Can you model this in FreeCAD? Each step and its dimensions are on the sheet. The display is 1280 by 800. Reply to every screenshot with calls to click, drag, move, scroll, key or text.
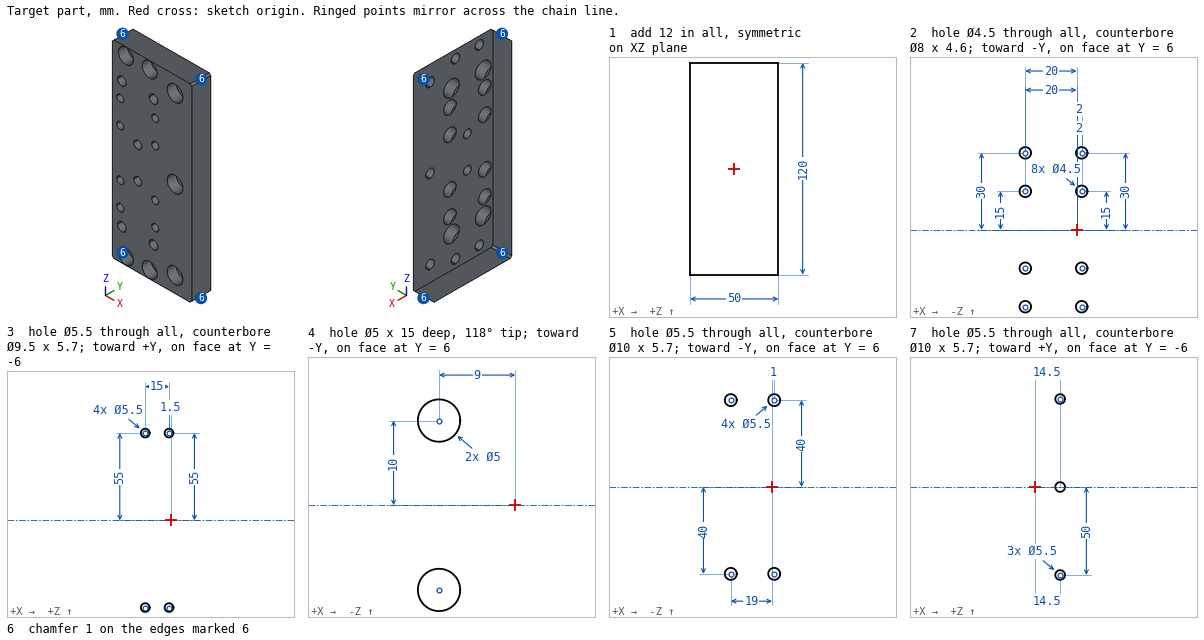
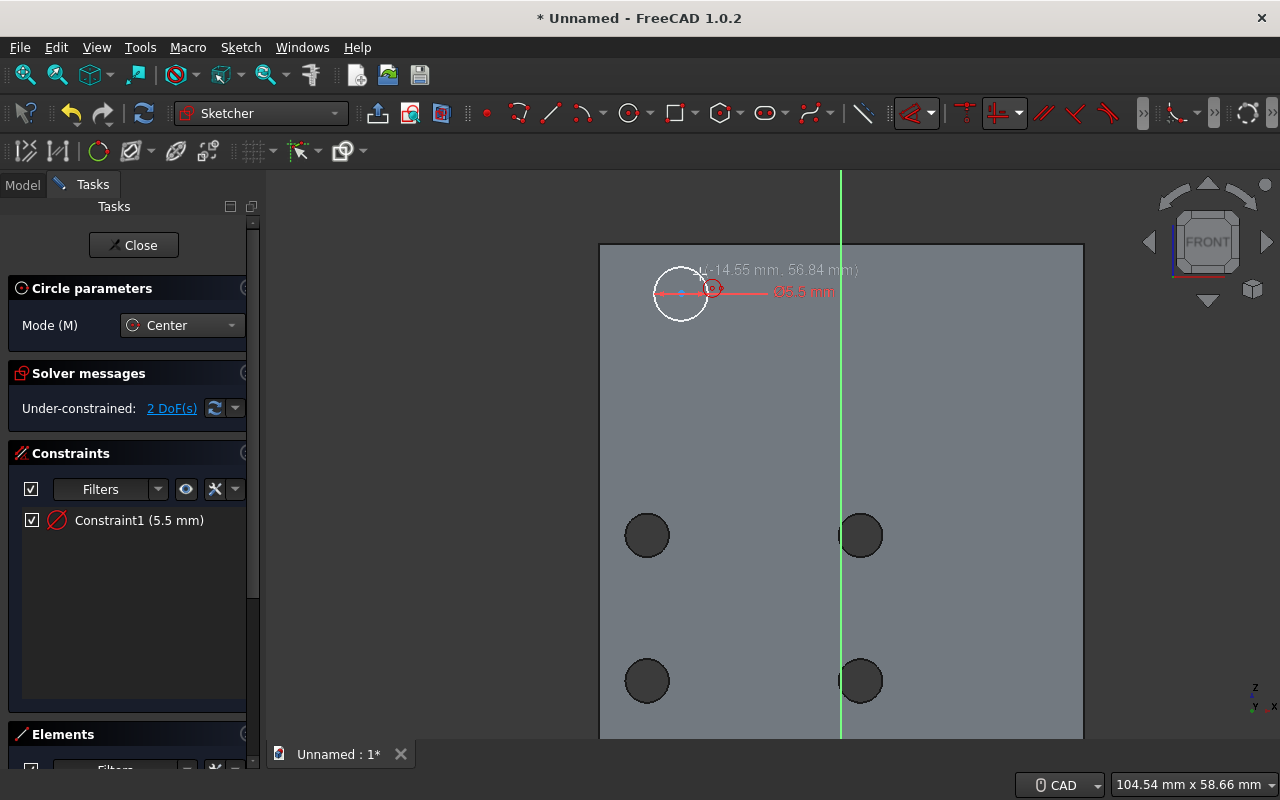
click(827, 293)
move(808, 274)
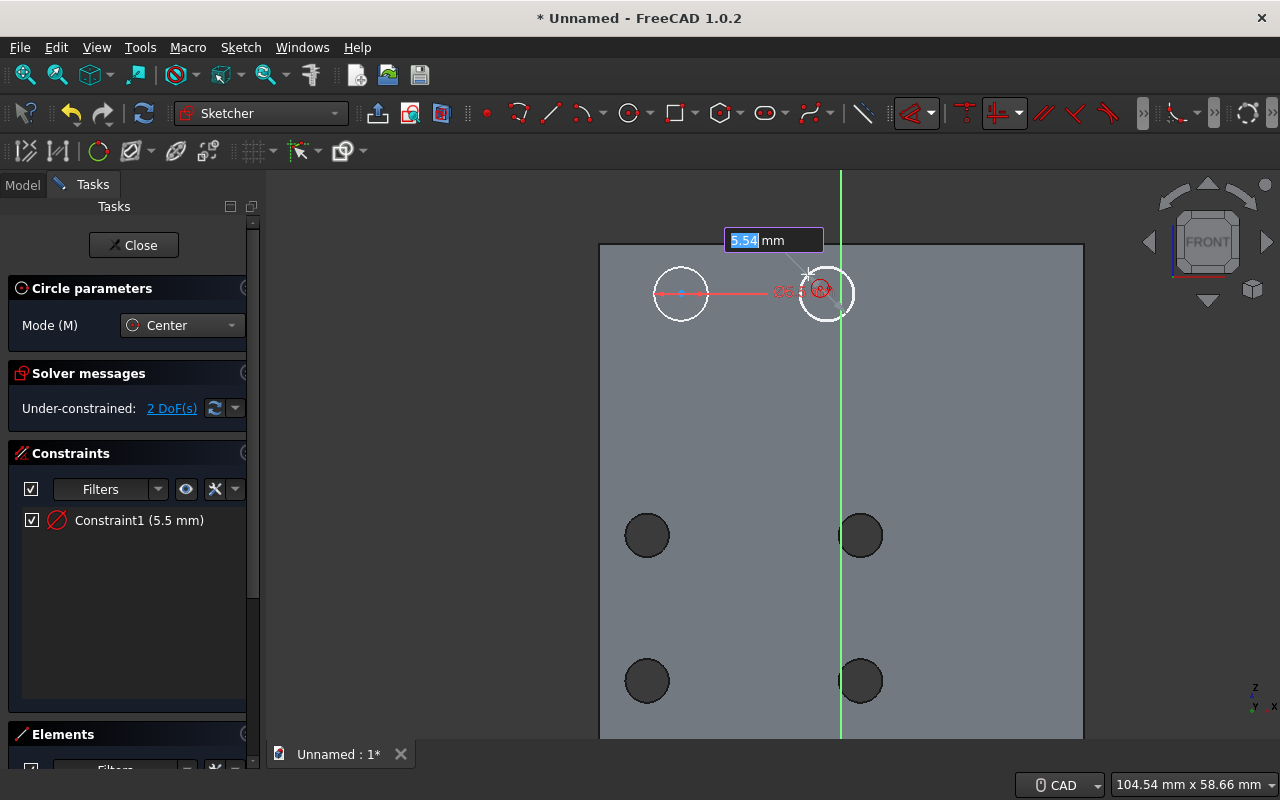
text(5.5)
key(Return)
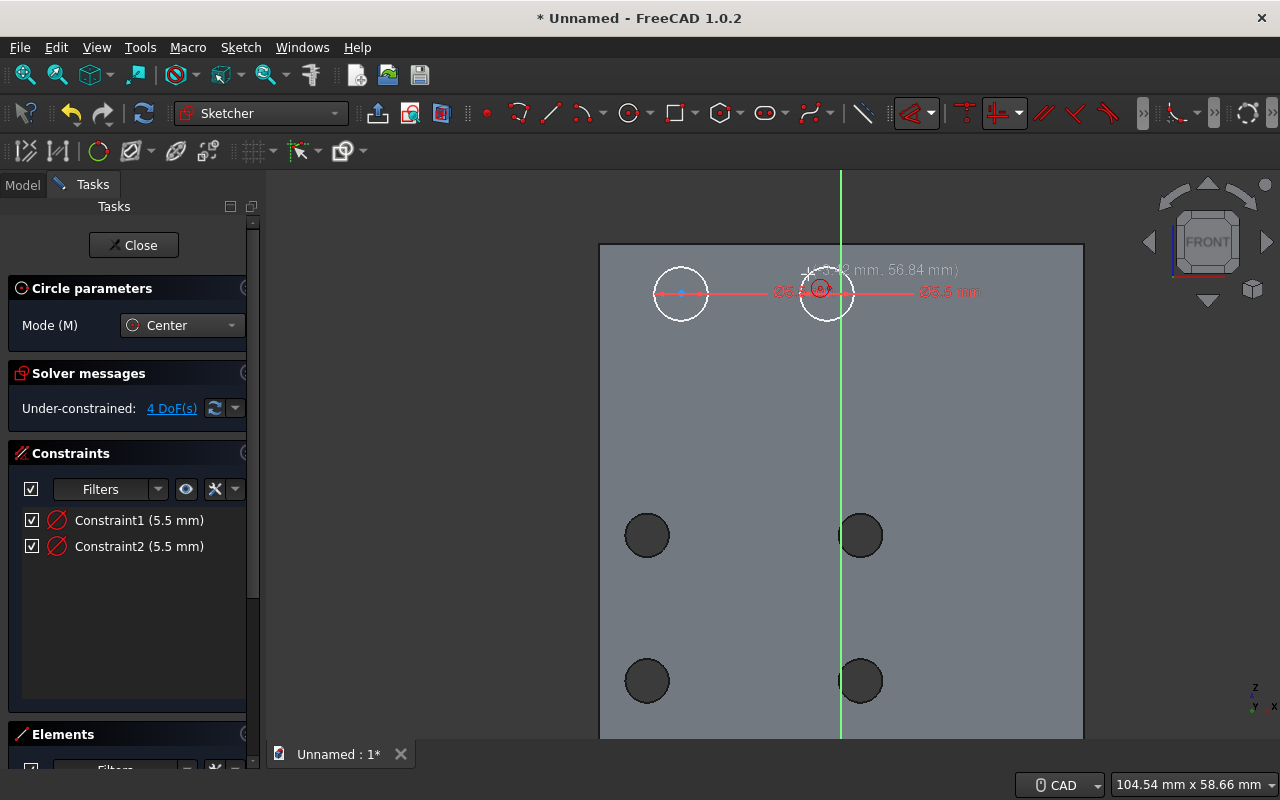
scroll(683, 294, down, 6)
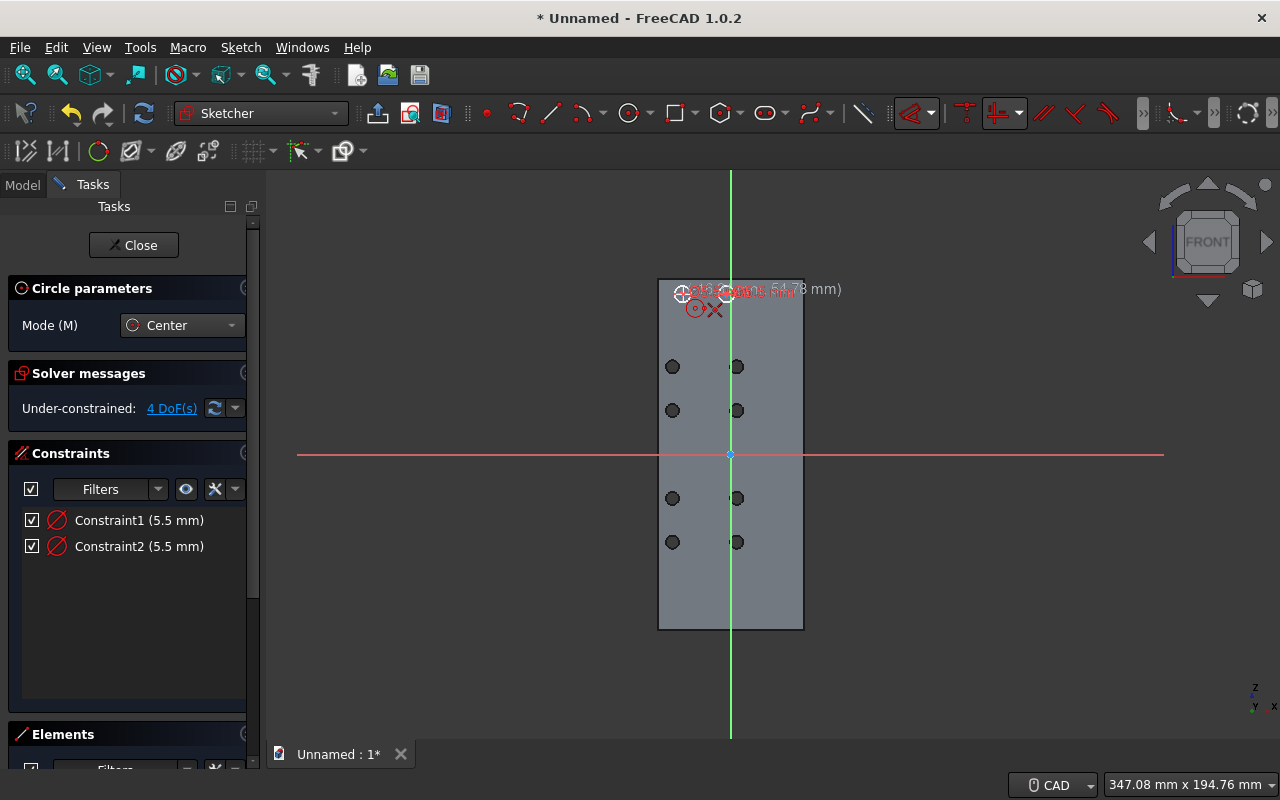
scroll(727, 615, up, 7)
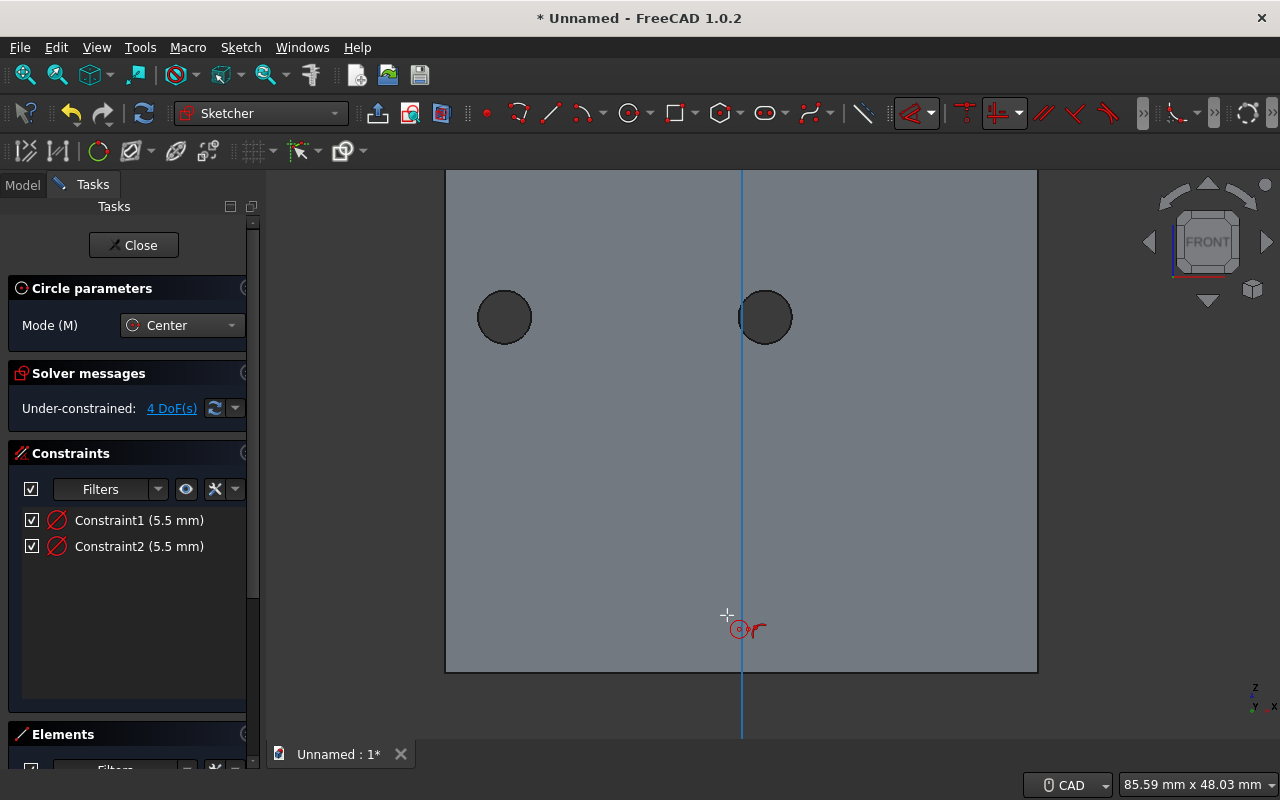
click(724, 613)
move(701, 590)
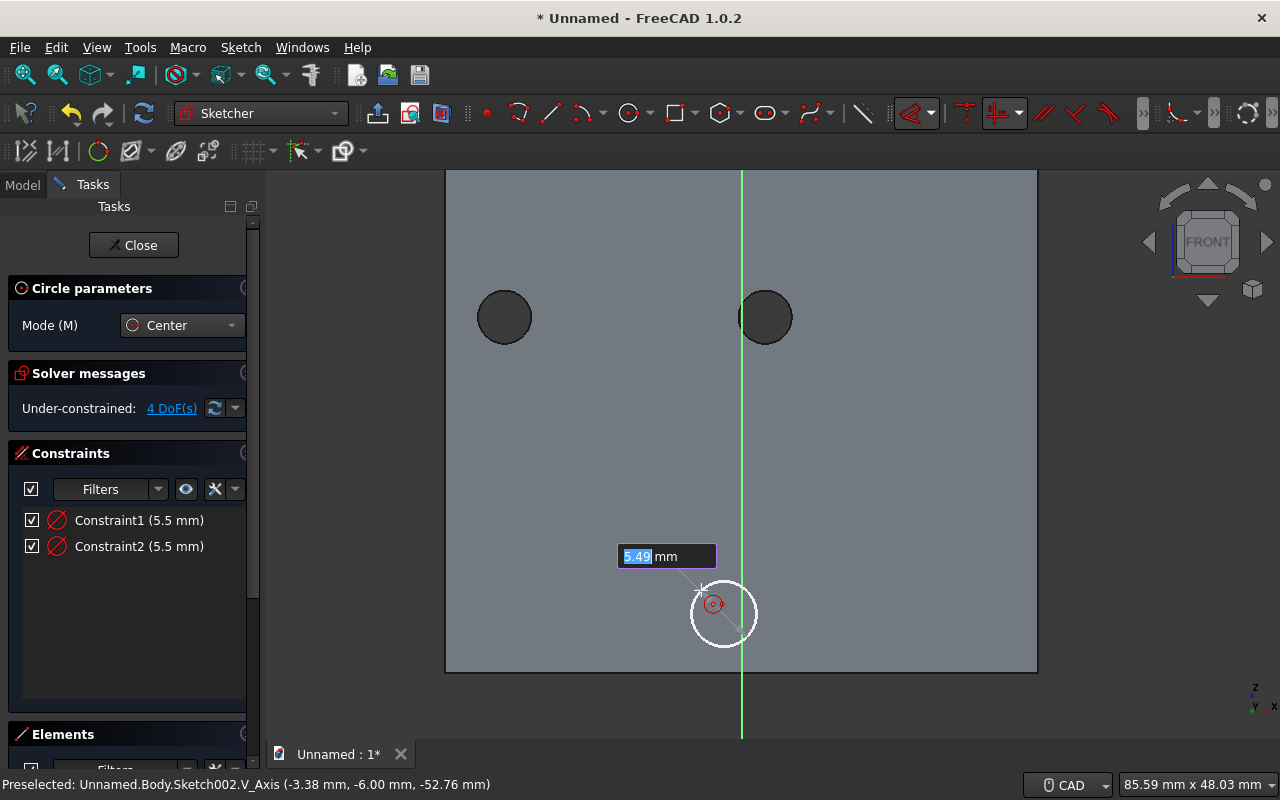
text(5.5)
key(Return)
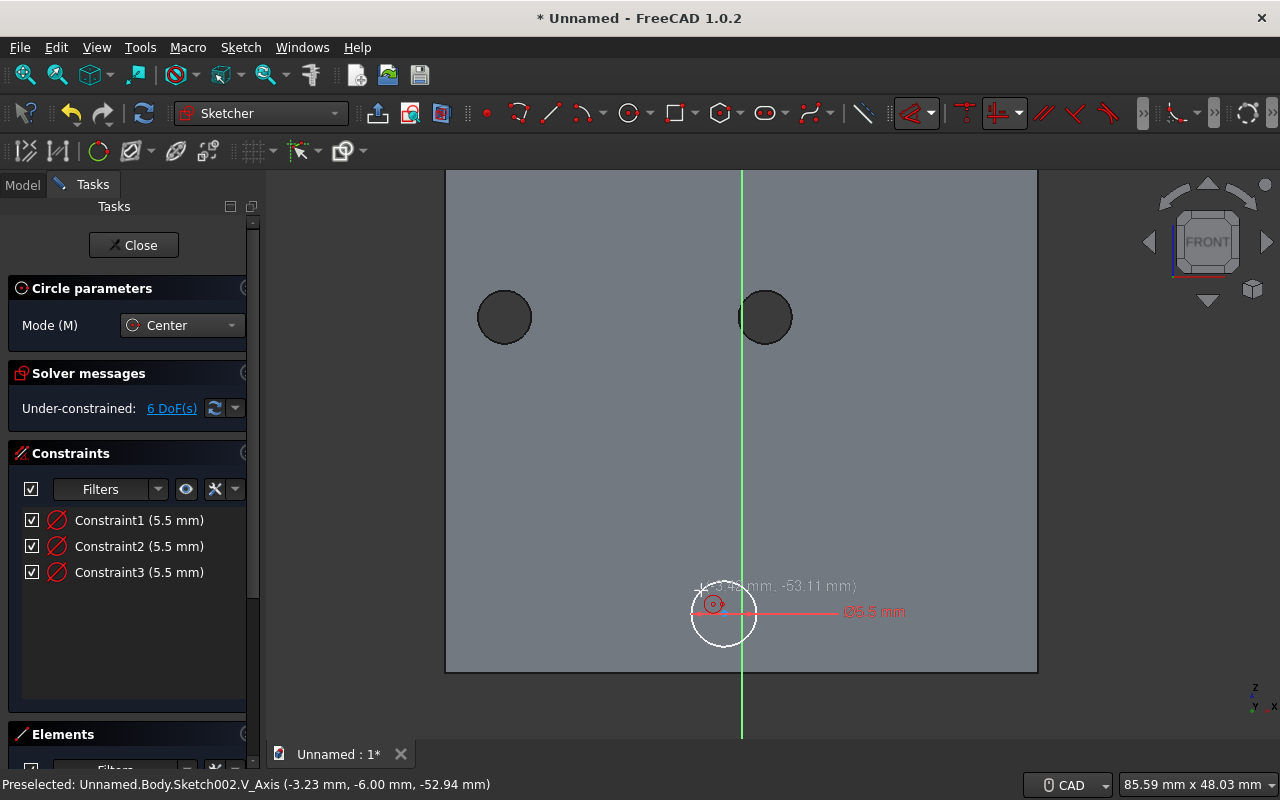
scroll(727, 616, down, 7)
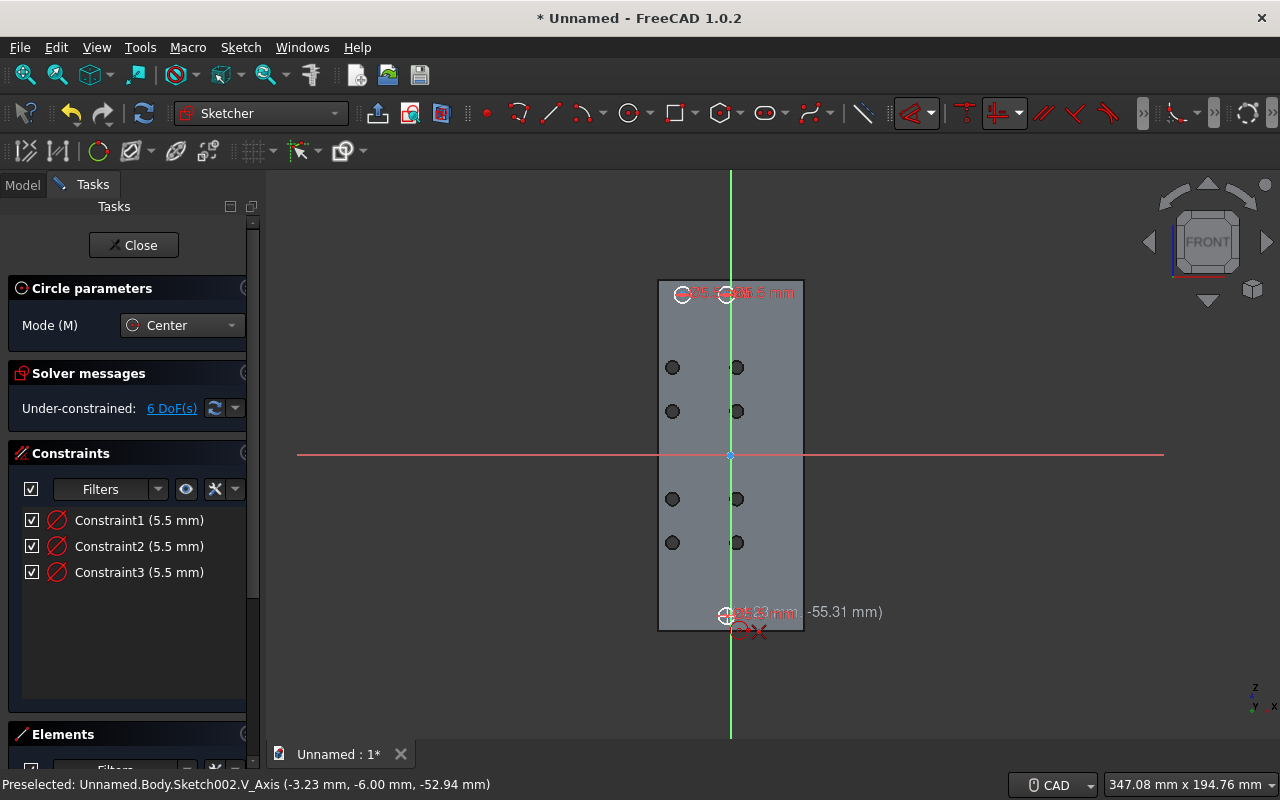
click(683, 616)
move(688, 610)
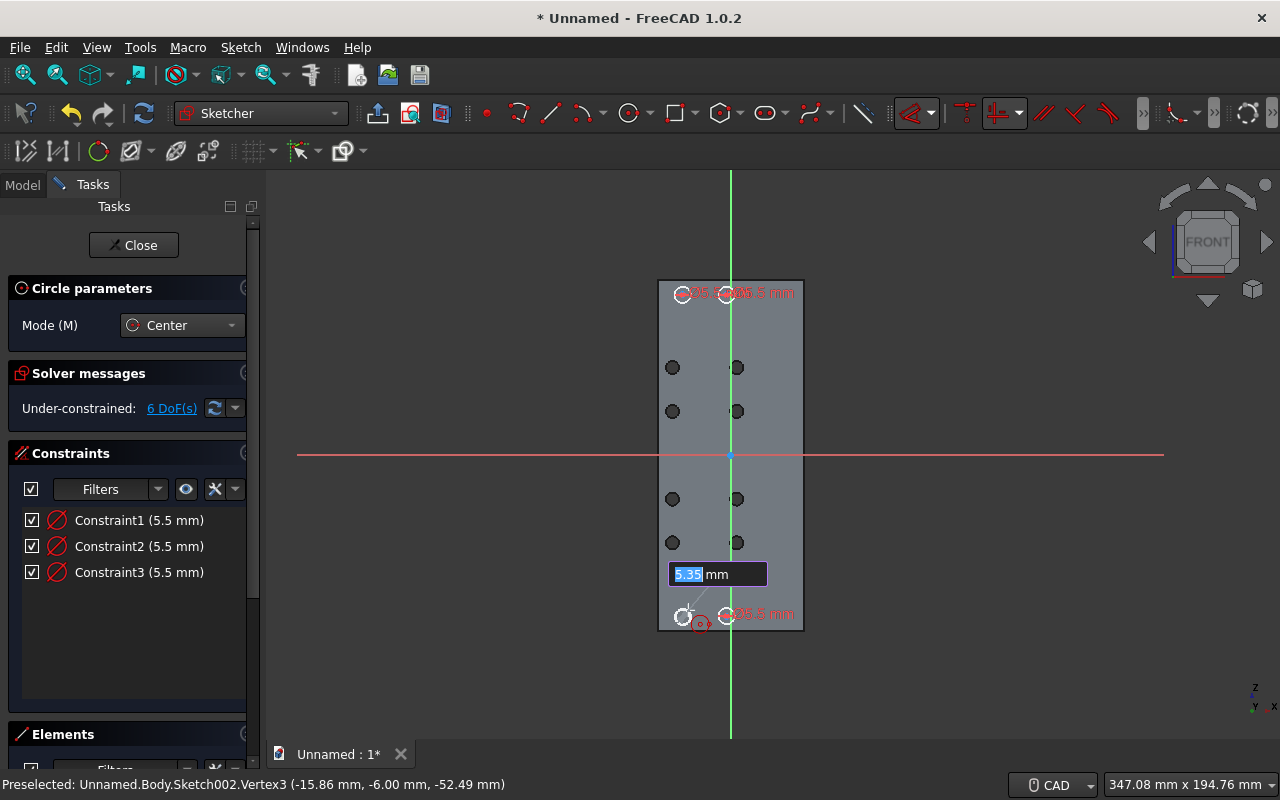
text(5.5)
key(Return)
key(Escape)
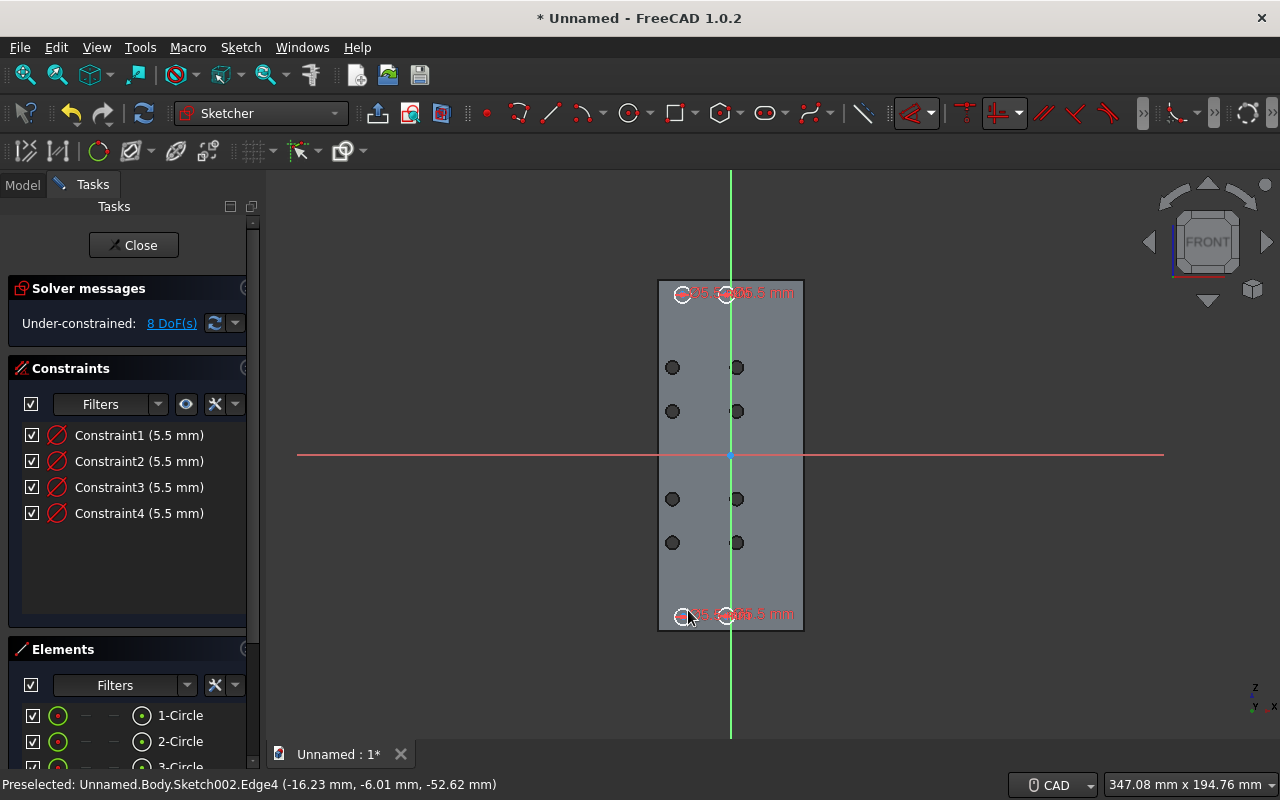
click(727, 295)